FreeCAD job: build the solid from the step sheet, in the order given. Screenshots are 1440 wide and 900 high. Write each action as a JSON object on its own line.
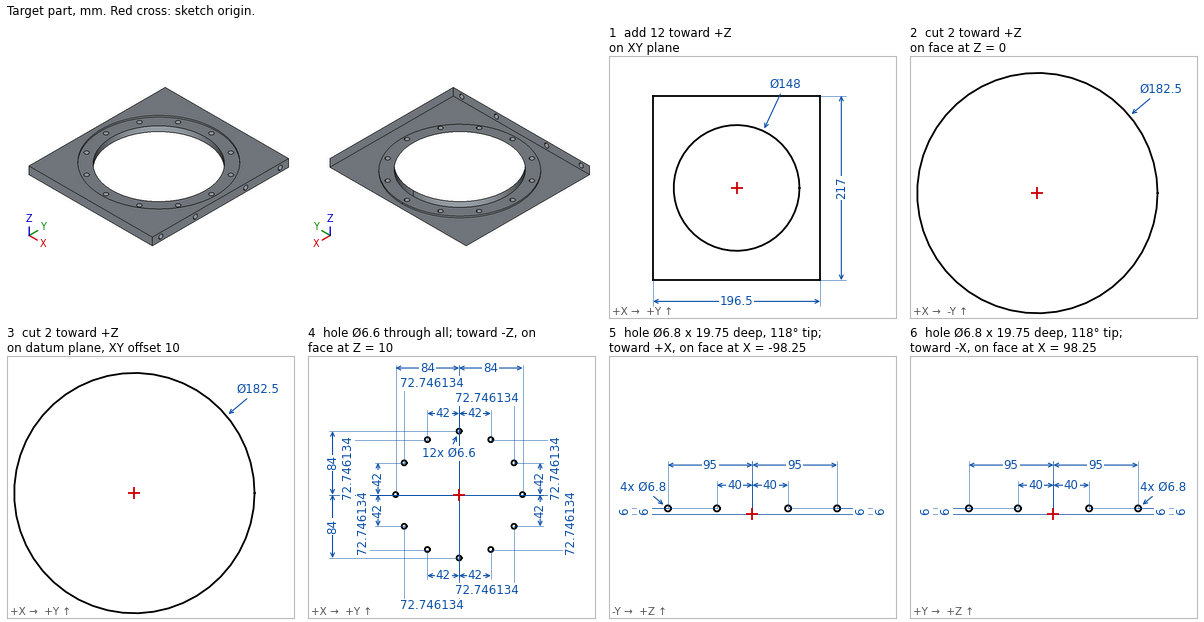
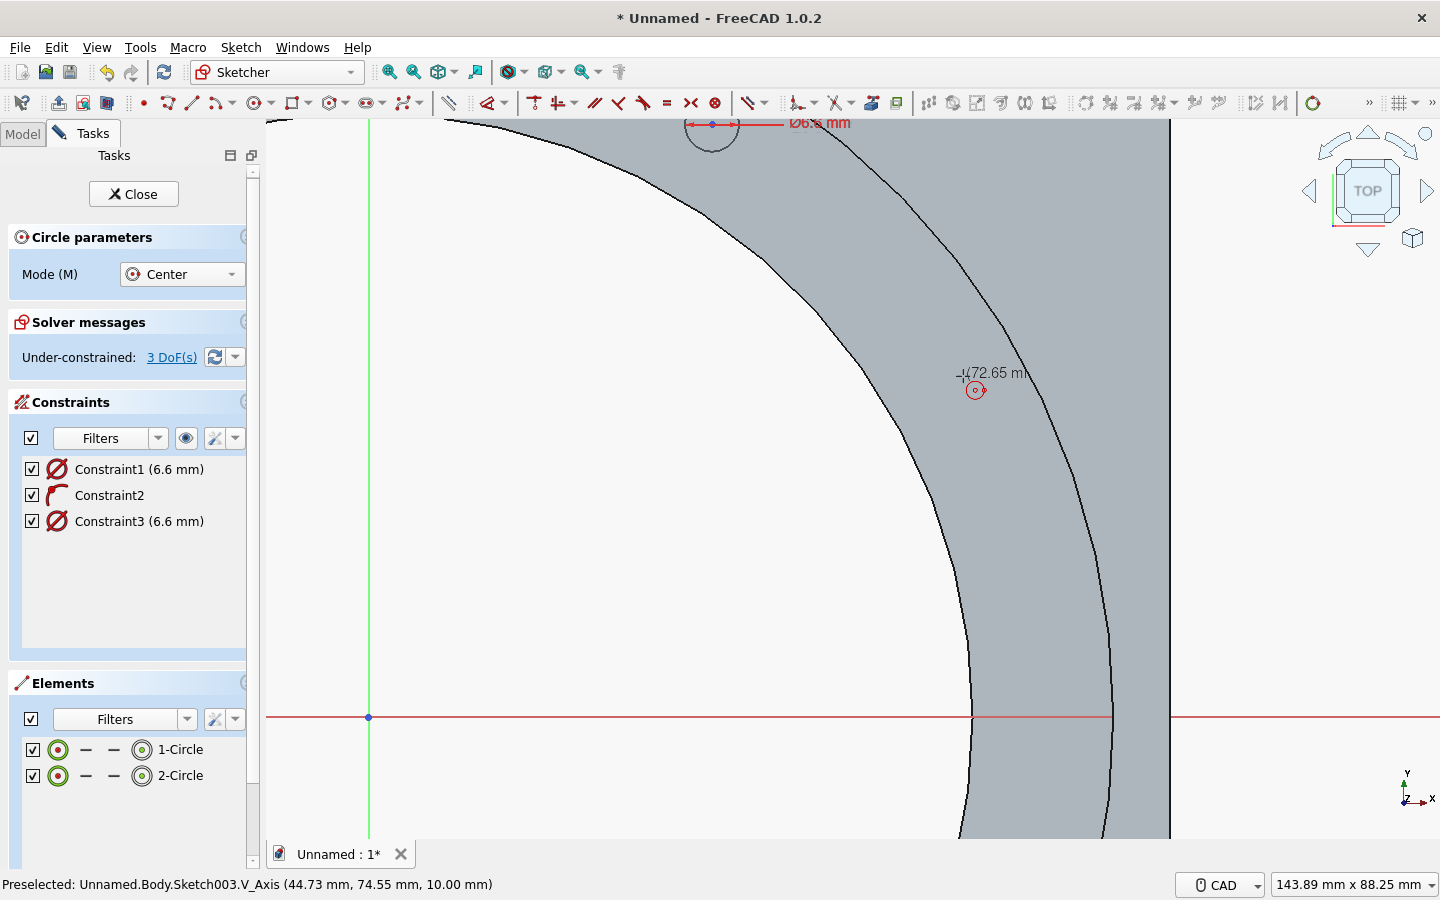
{"action": "left_click", "coordinate": [962, 374]}
{"action": "mouse_move", "coordinate": [981, 355]}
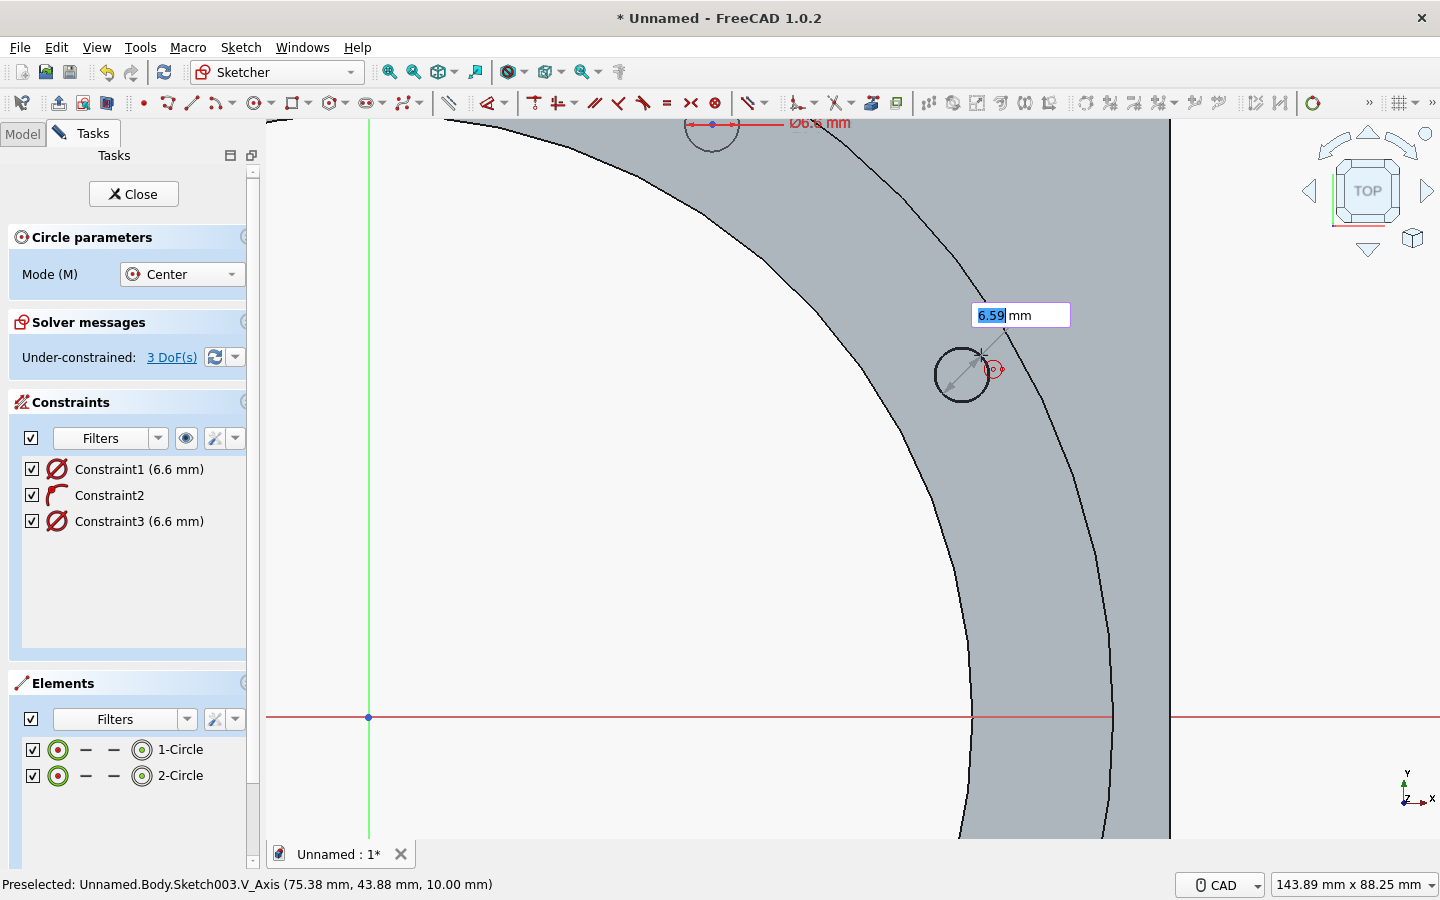
{"action": "type", "text": "6.6"}
{"action": "key", "text": "Return"}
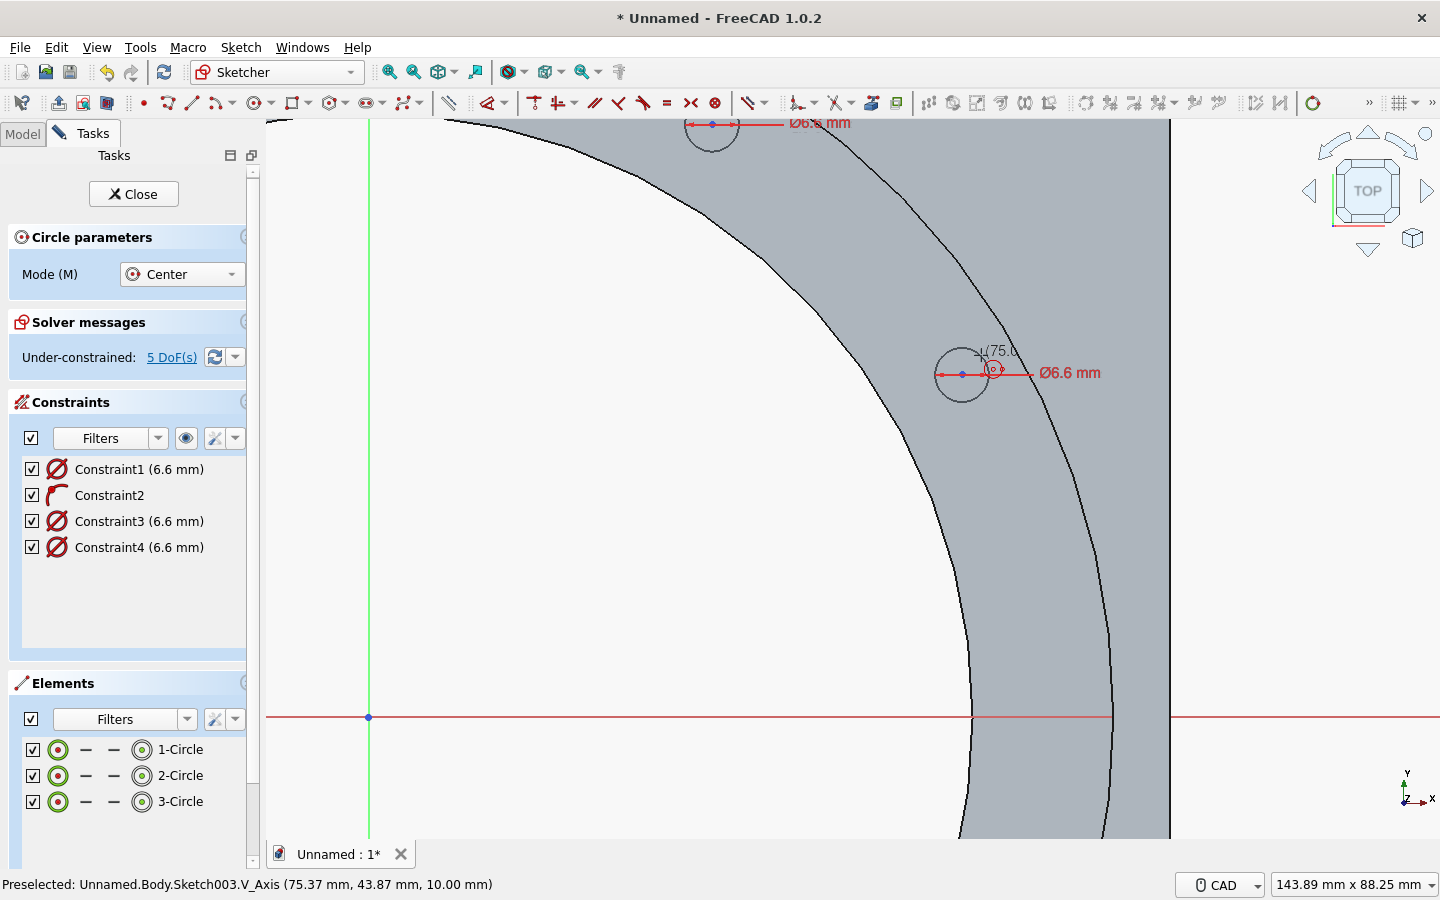
{"action": "left_click", "coordinate": [1054, 717]}
{"action": "mouse_move", "coordinate": [1073, 698]}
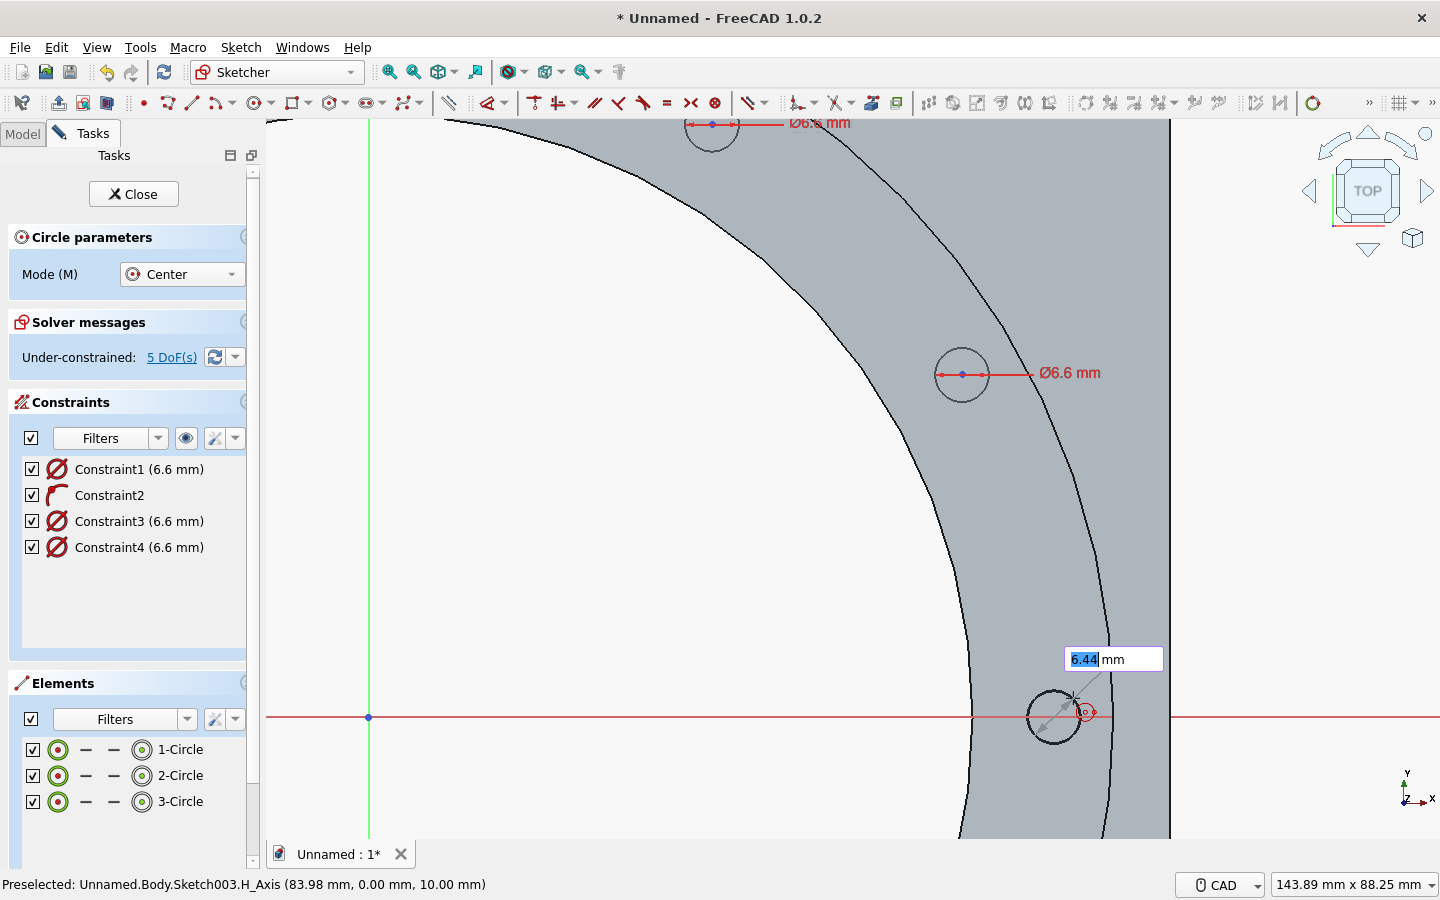
{"action": "type", "text": "6.6"}
{"action": "key", "text": "Return"}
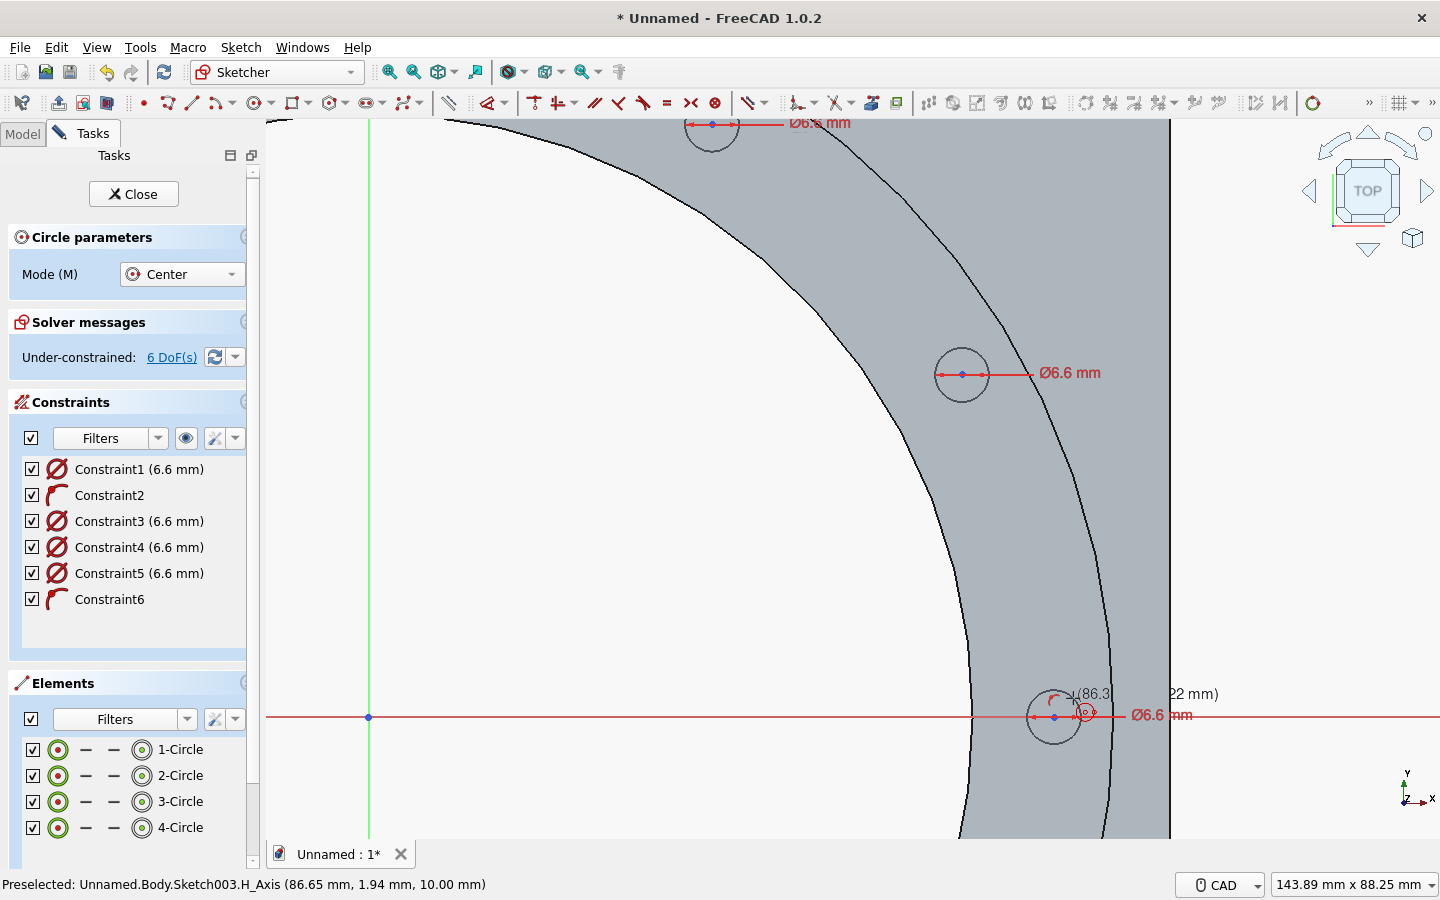
{"action": "scroll", "coordinate": [964, 376], "scroll_direction": "down", "scroll_amount": 6}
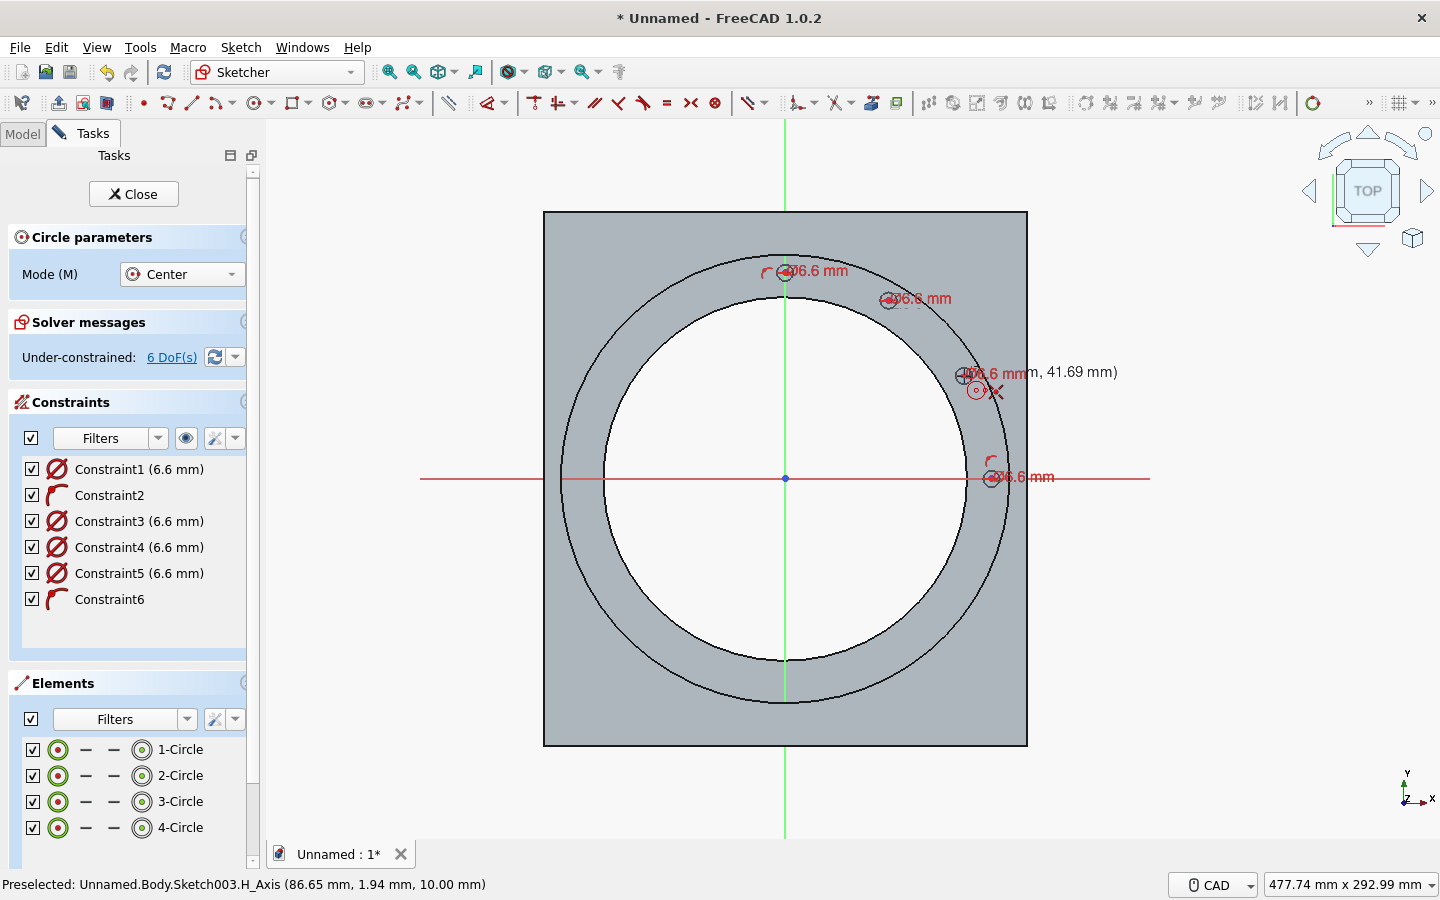
{"action": "scroll", "coordinate": [964, 582], "scroll_direction": "up", "scroll_amount": 6}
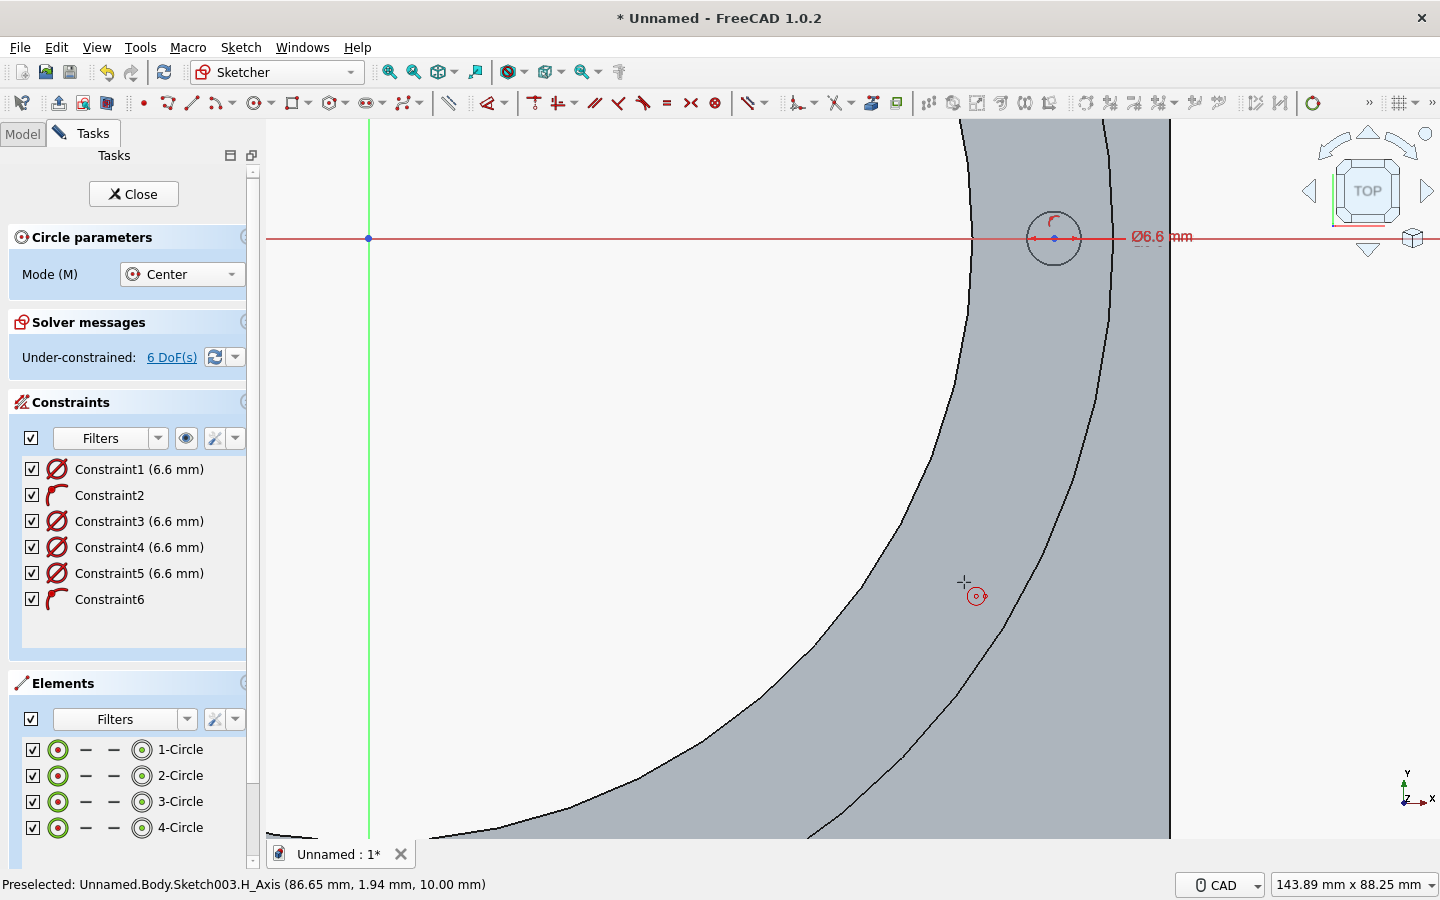
{"action": "left_click", "coordinate": [962, 581]}
{"action": "mouse_move", "coordinate": [981, 562]}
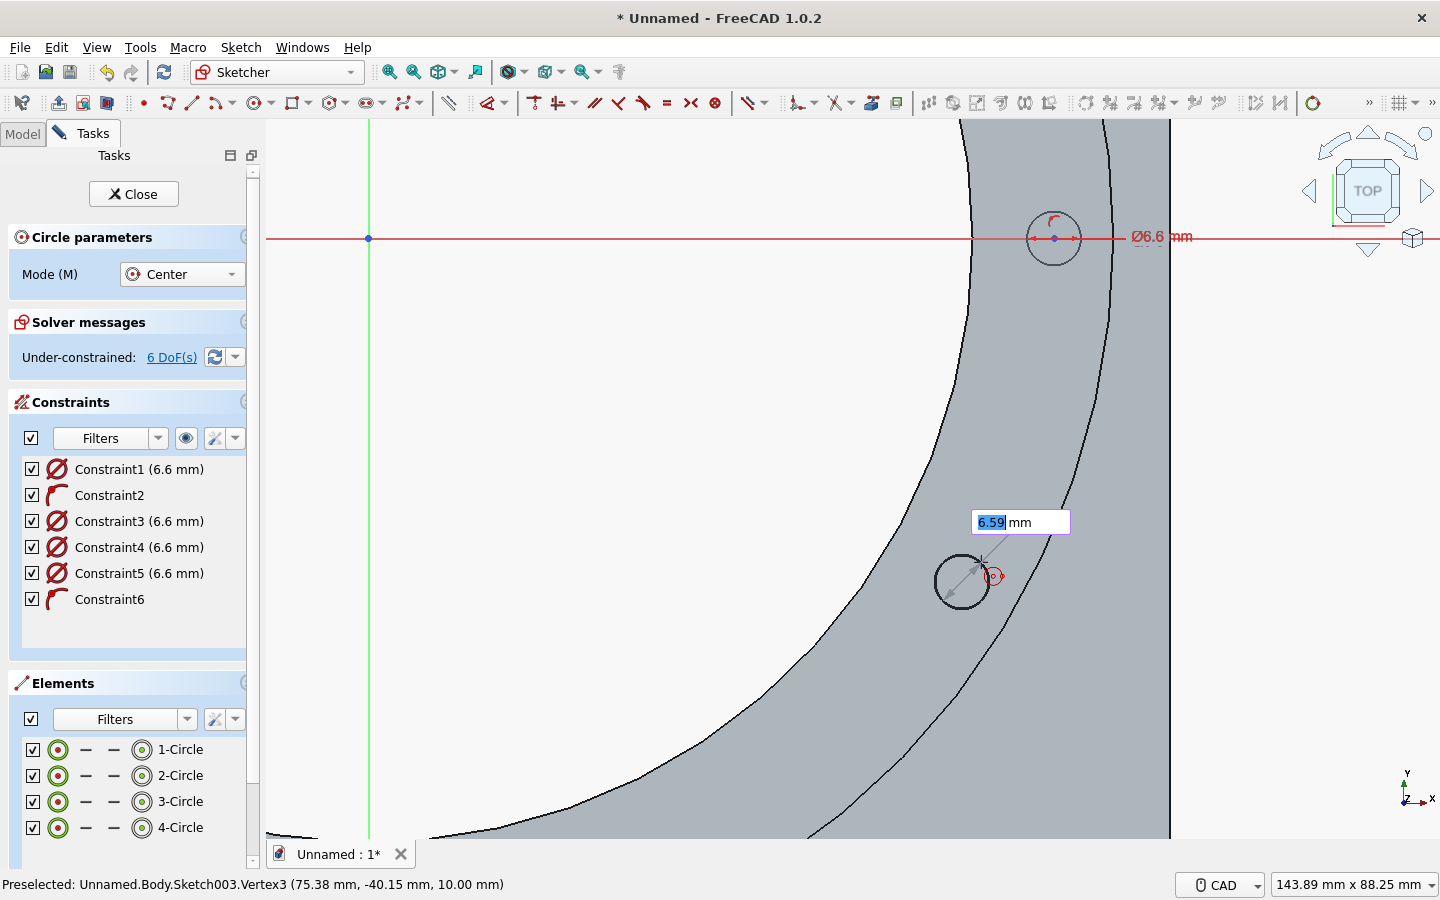
{"action": "type", "text": "6.6"}
{"action": "key", "text": "Return"}